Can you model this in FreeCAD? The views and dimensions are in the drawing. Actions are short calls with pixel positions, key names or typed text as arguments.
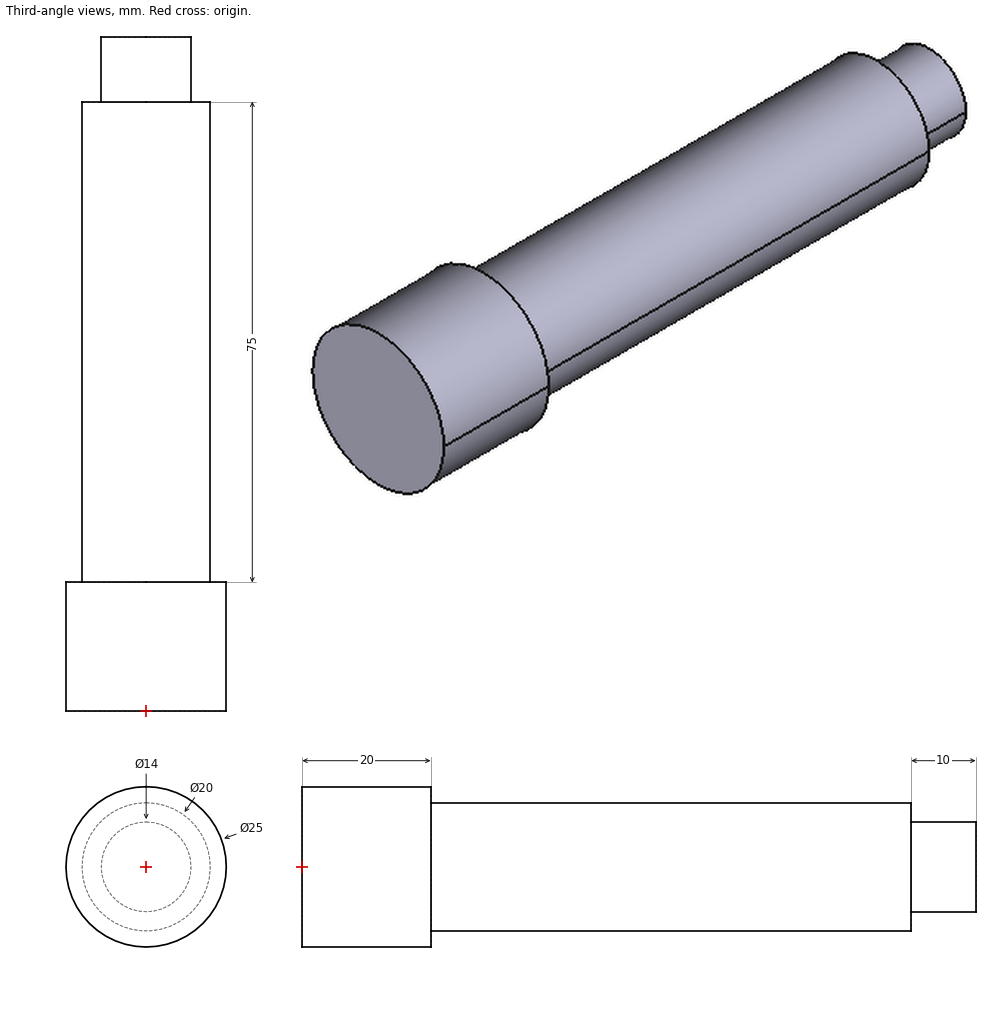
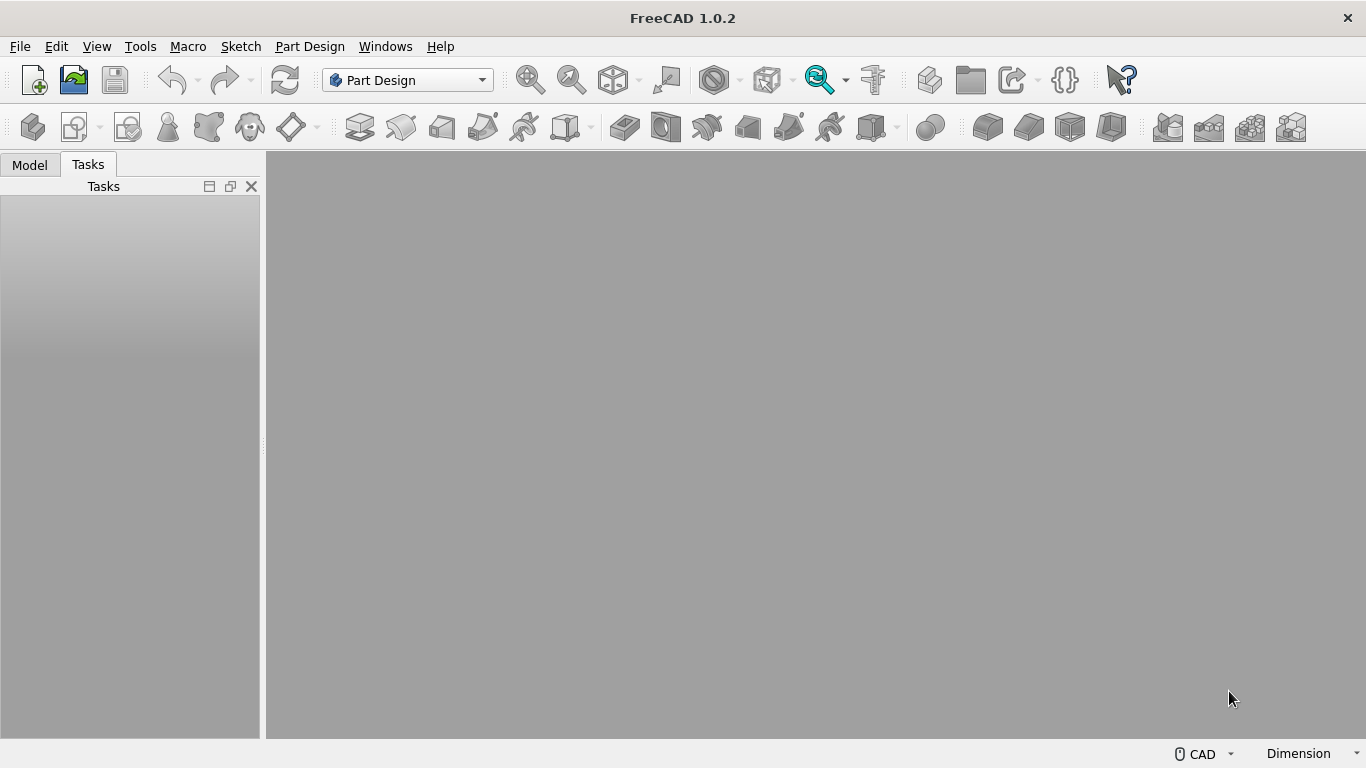
click(33, 80)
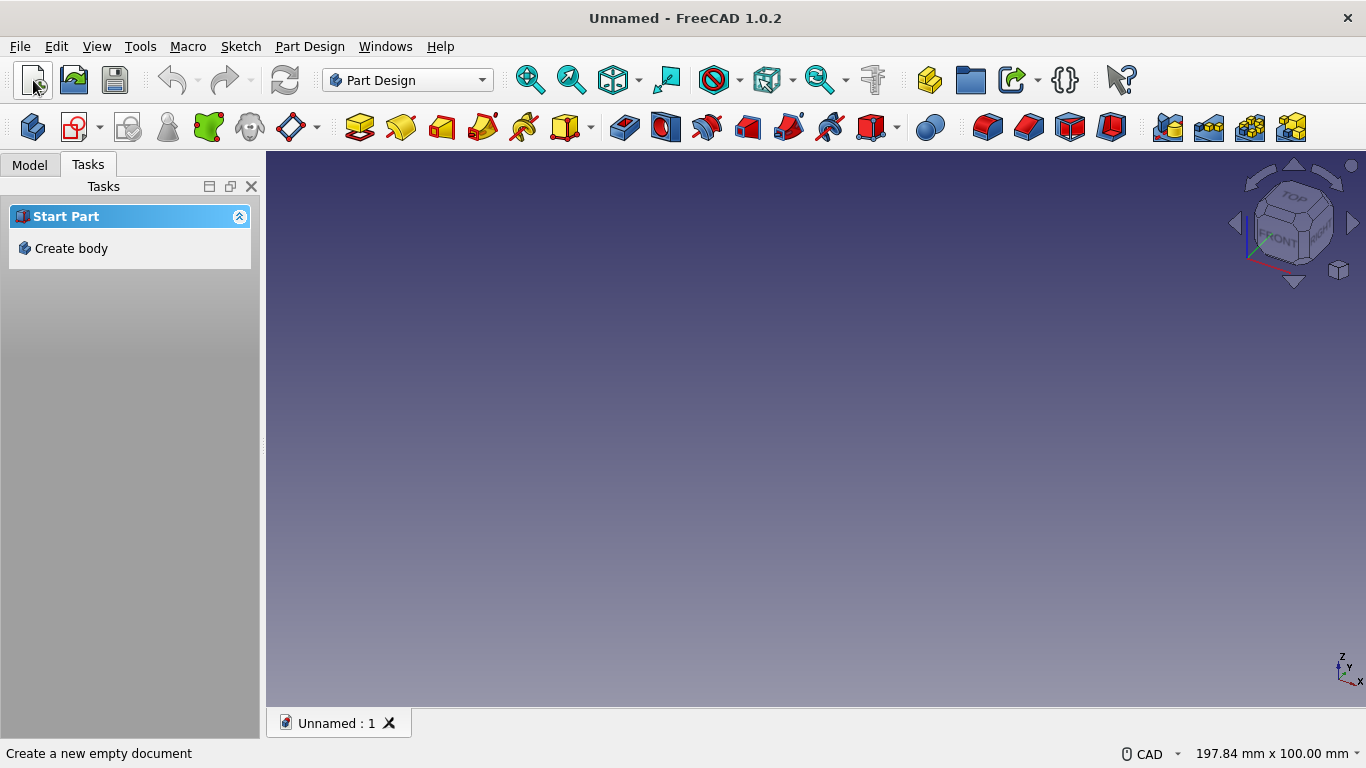
click(74, 128)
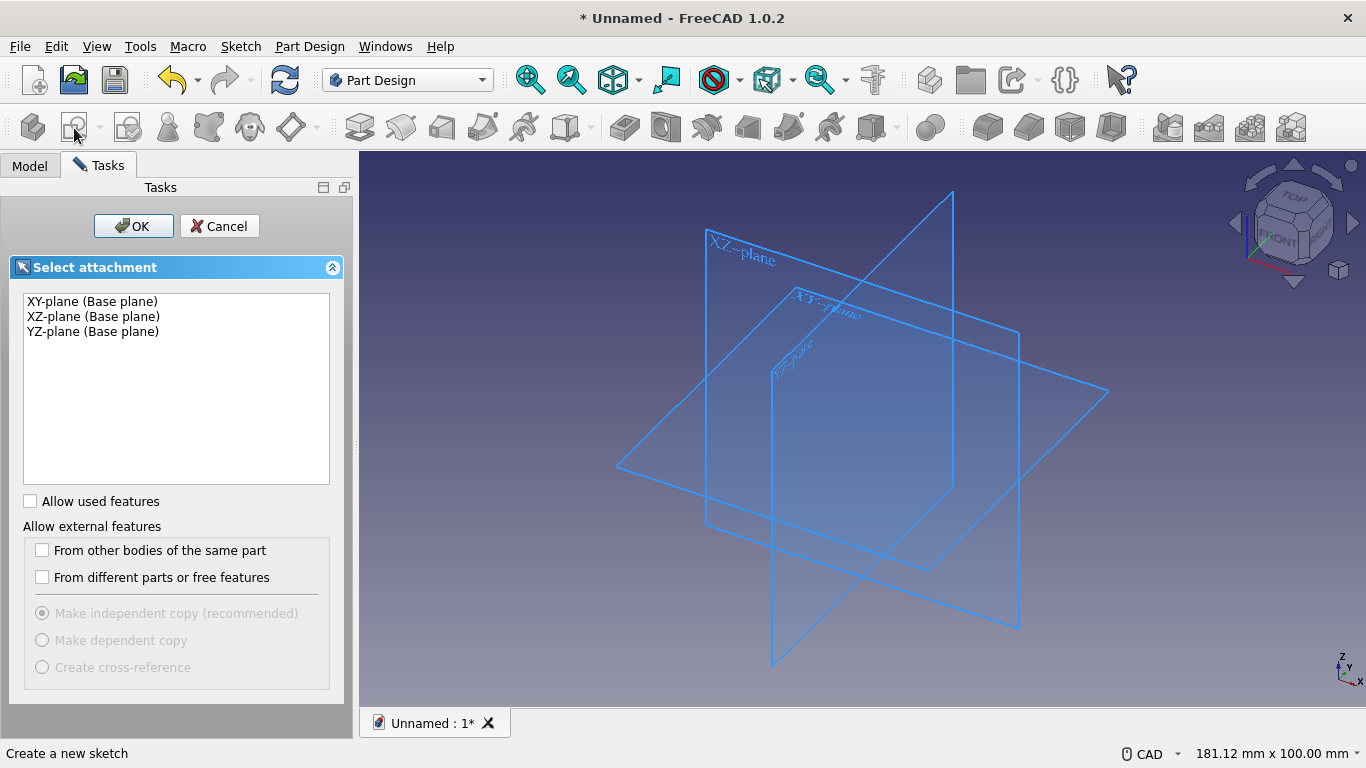
click(84, 316)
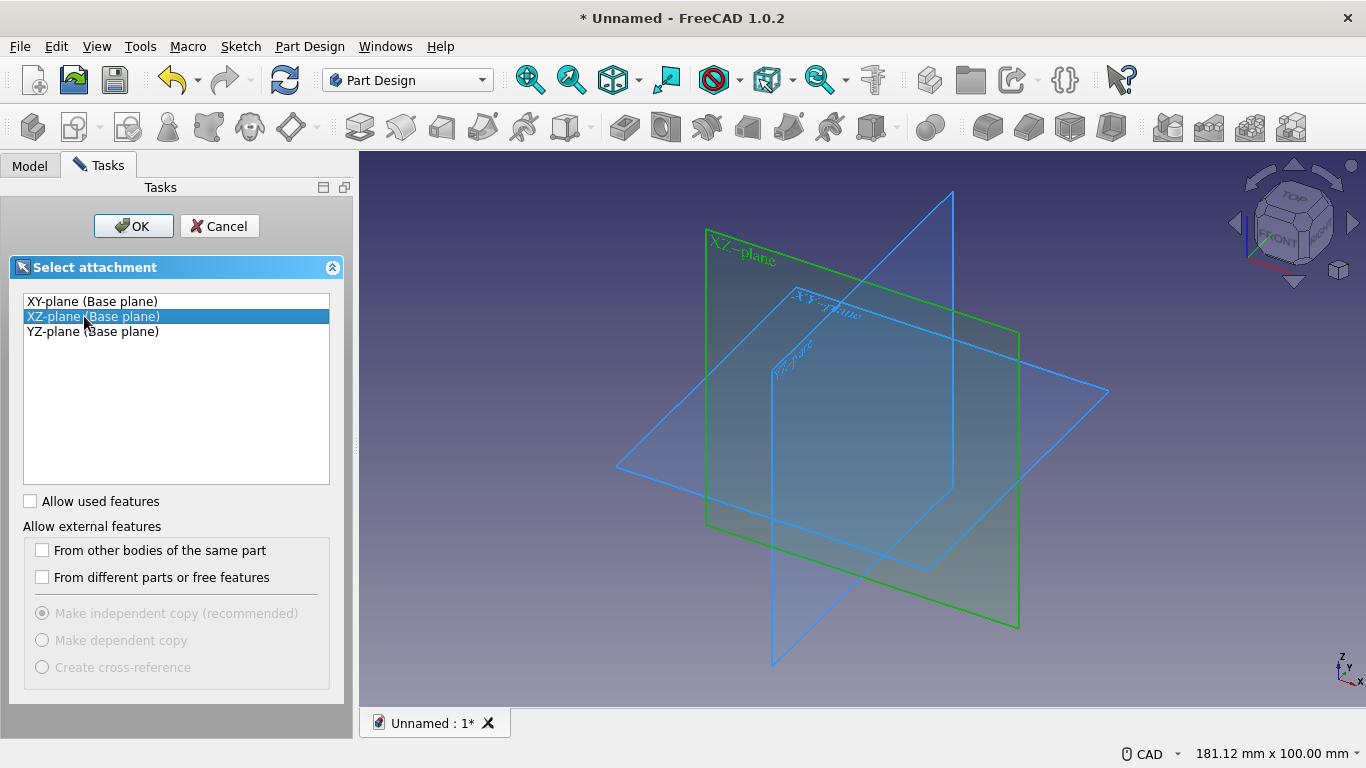
click(134, 226)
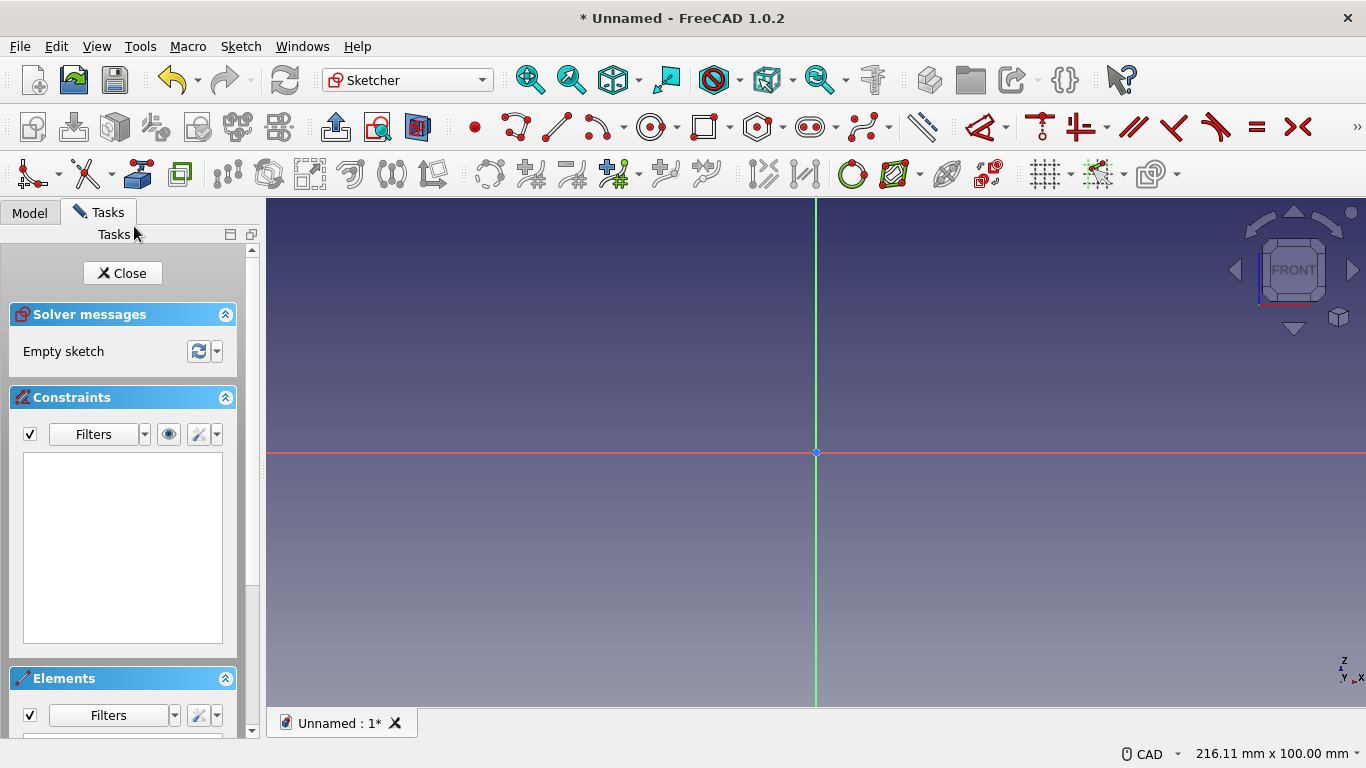
scroll(856, 453, up, 5)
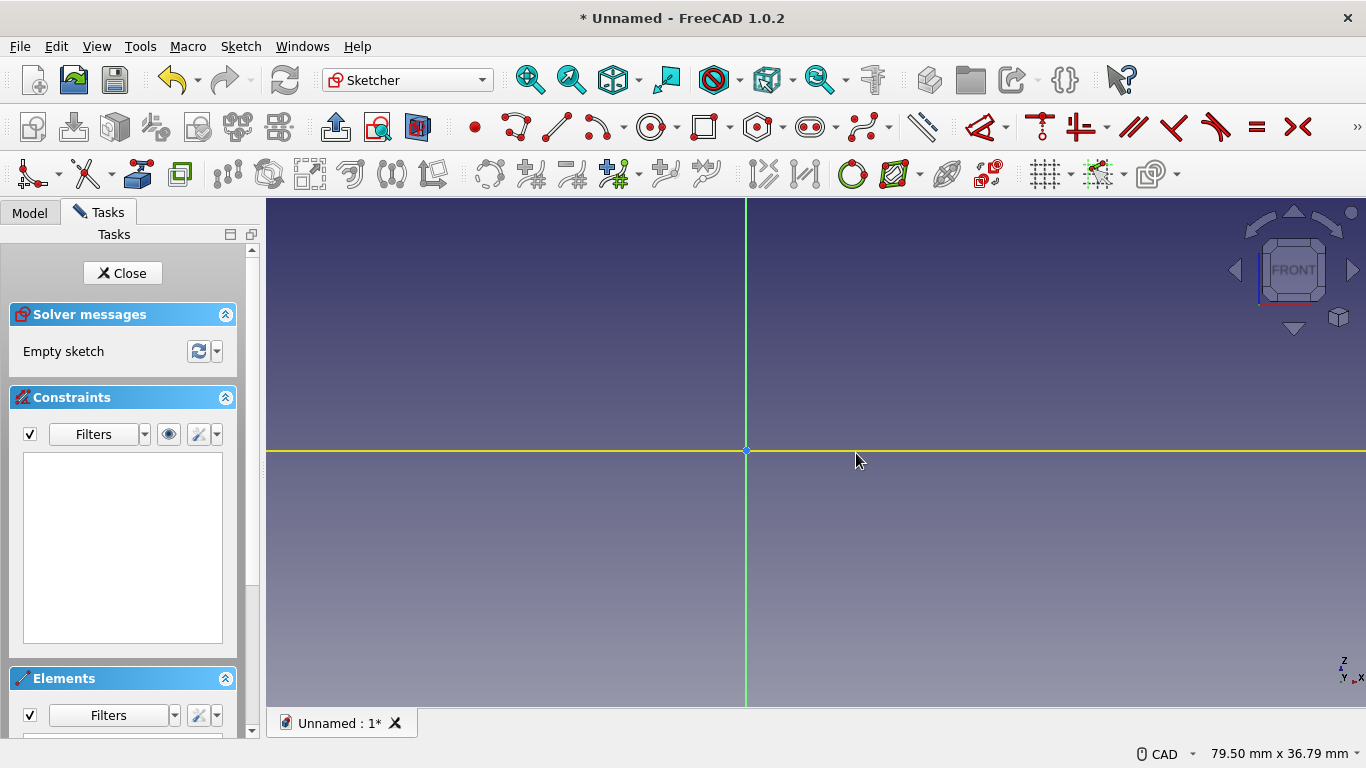
click(650, 128)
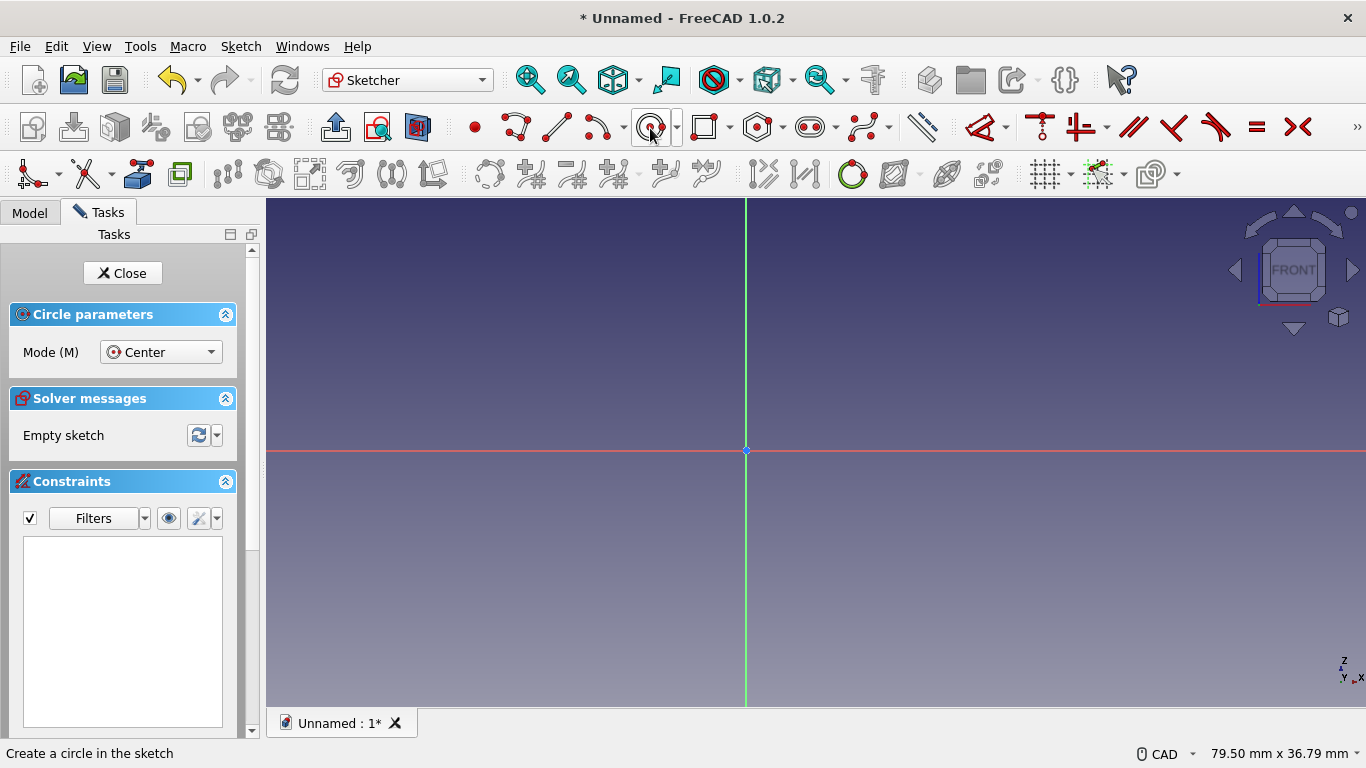
click(746, 451)
move(869, 328)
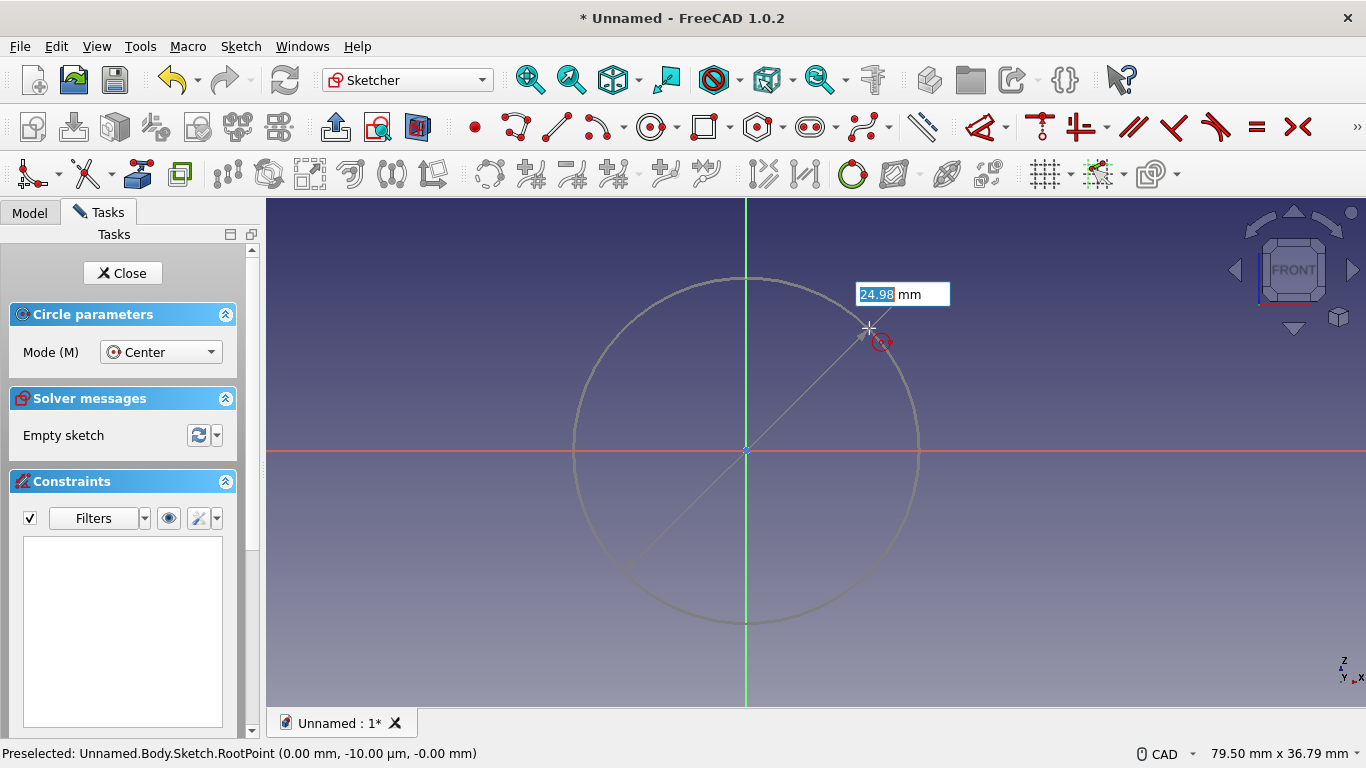
text(25)
key(Return)
key(Escape)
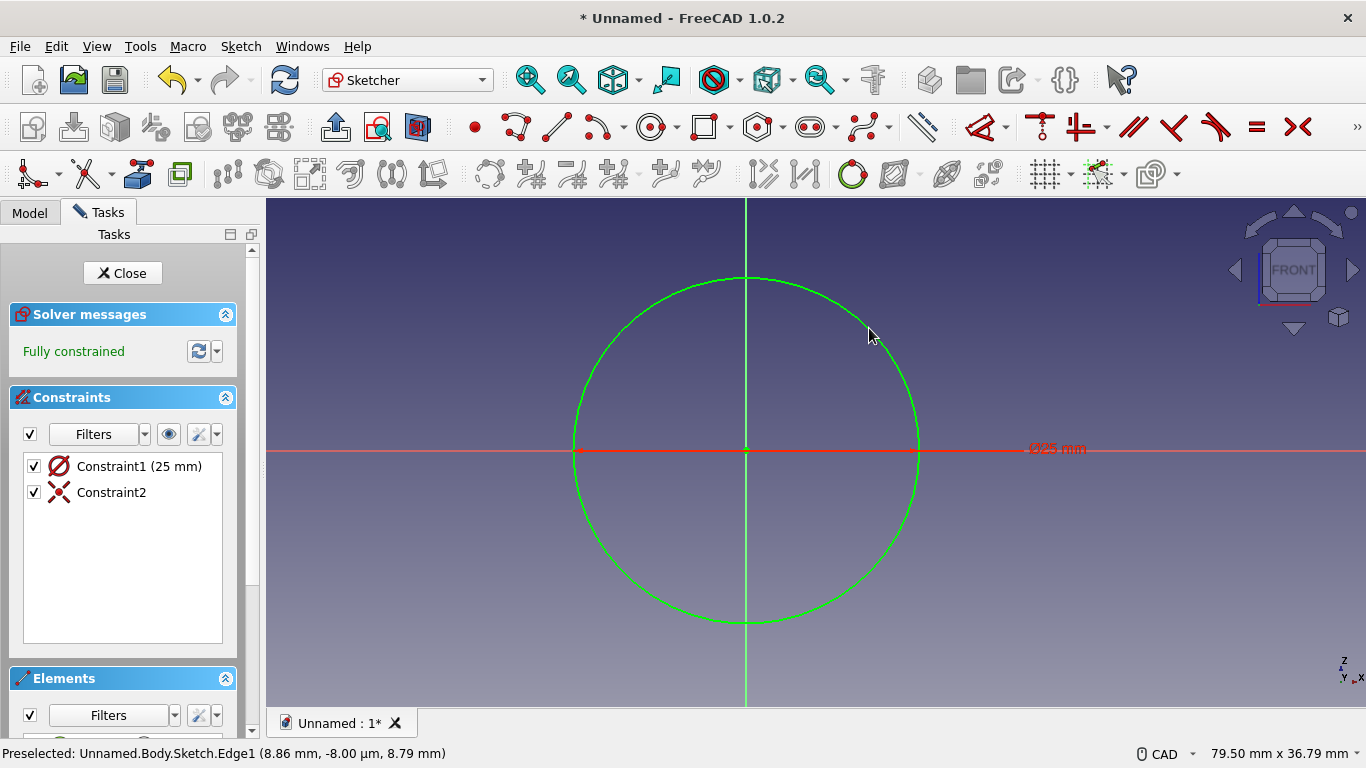
click(123, 273)